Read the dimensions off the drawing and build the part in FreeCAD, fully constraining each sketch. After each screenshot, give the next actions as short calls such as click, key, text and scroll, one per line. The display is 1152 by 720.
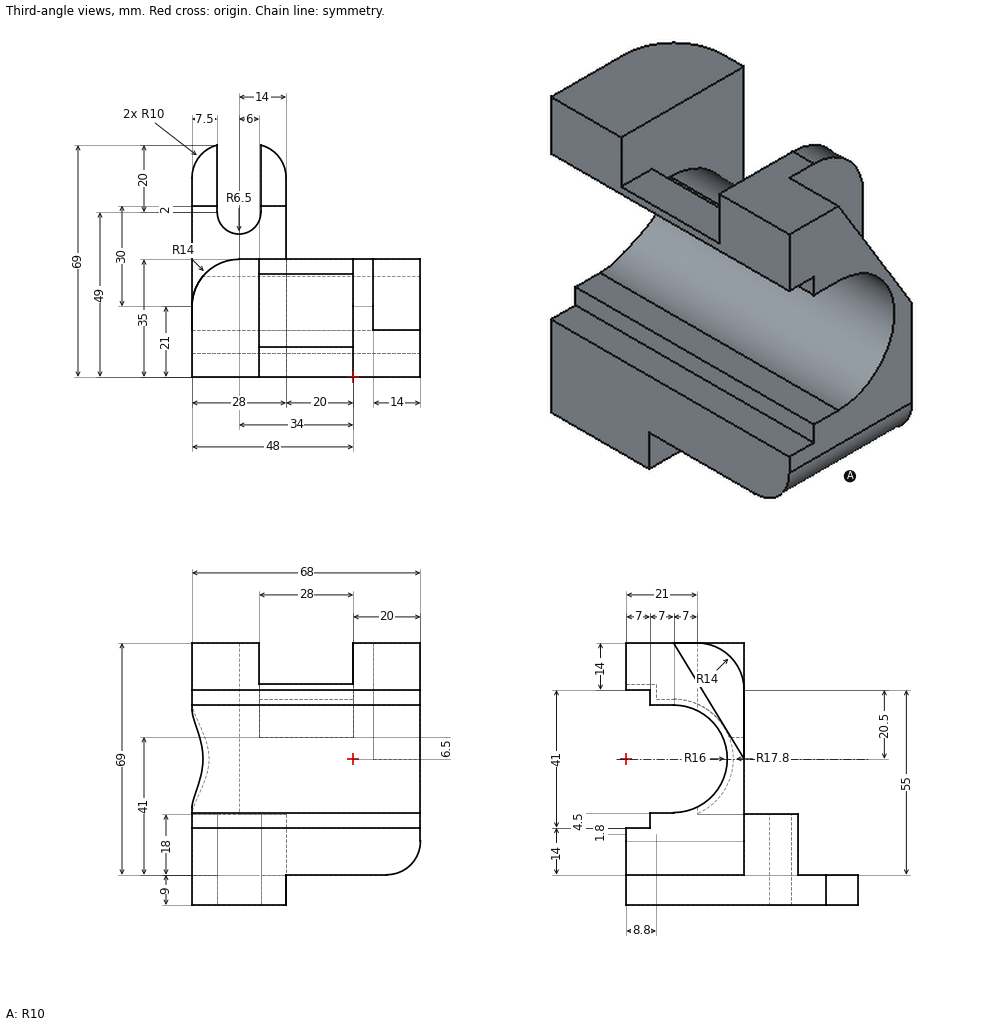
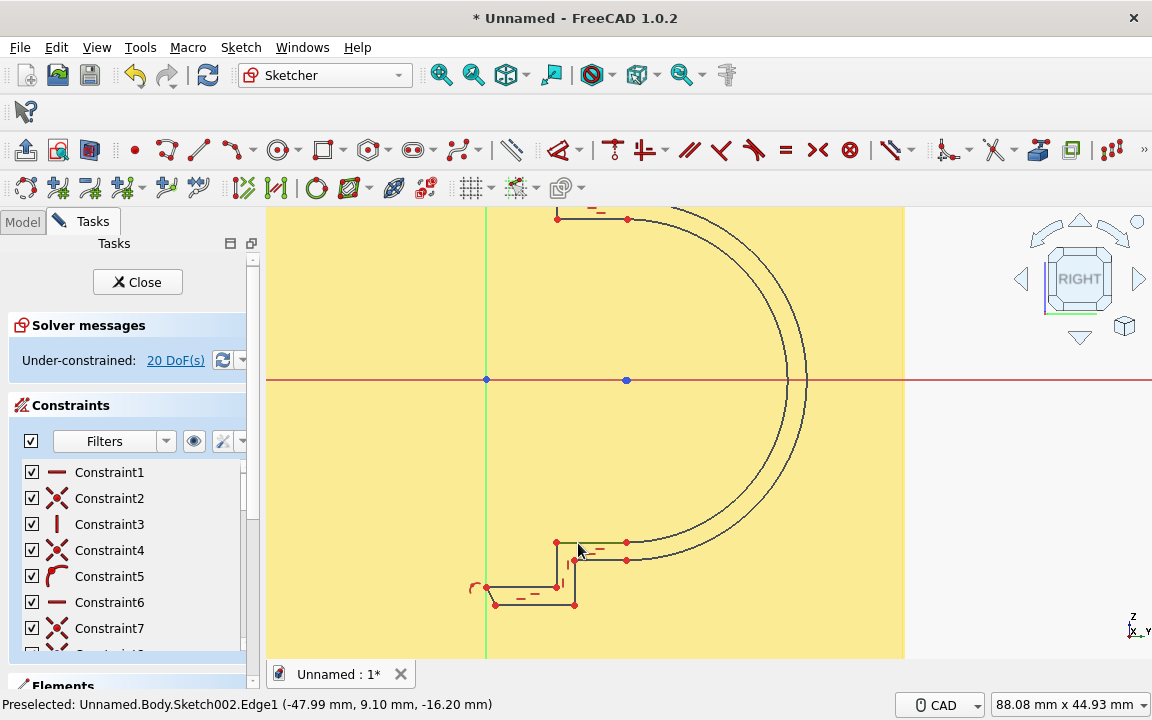
click(757, 476)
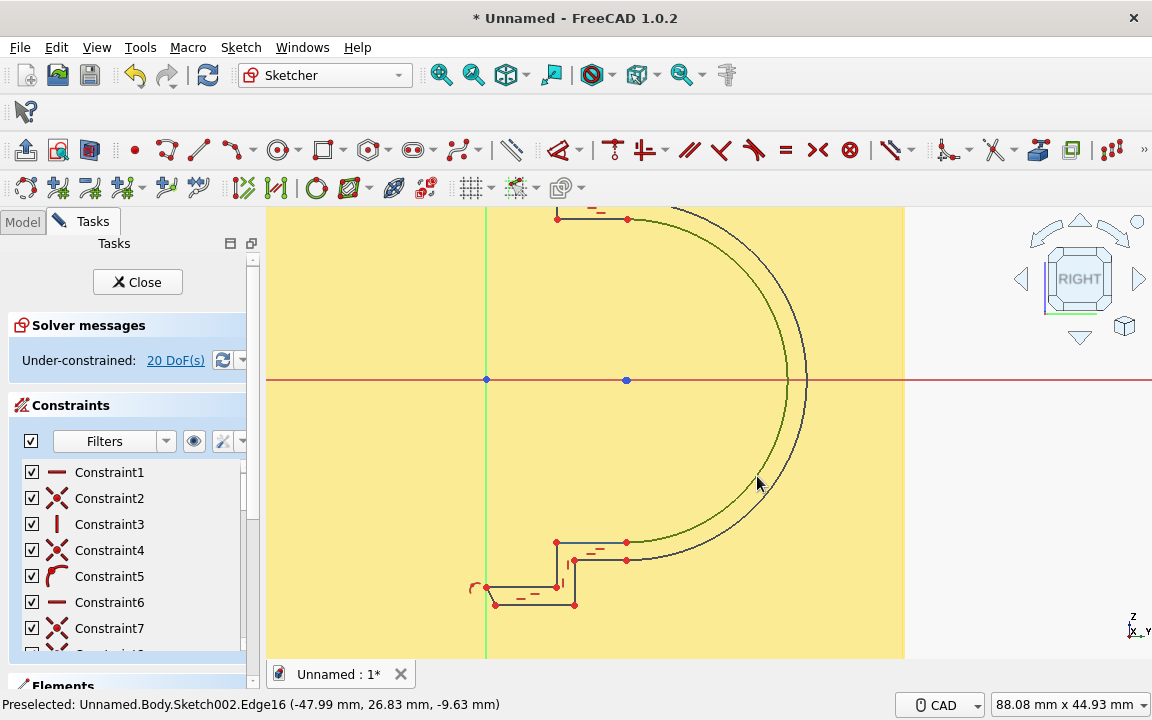
key(t)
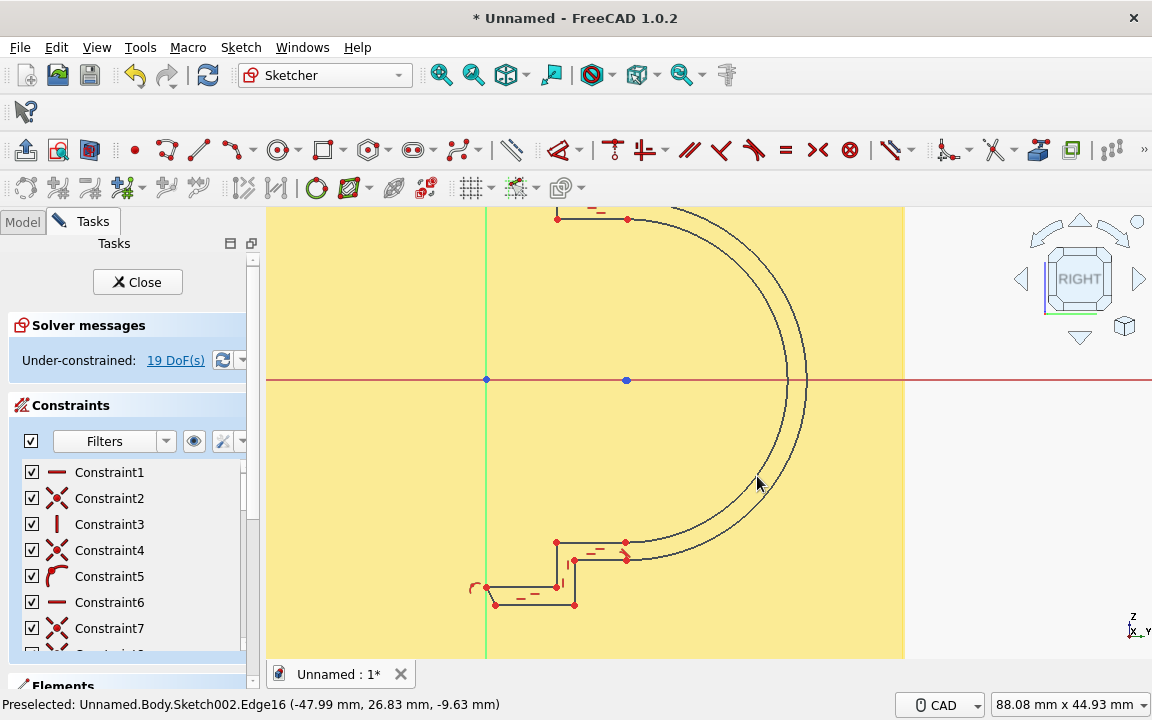
click(590, 560)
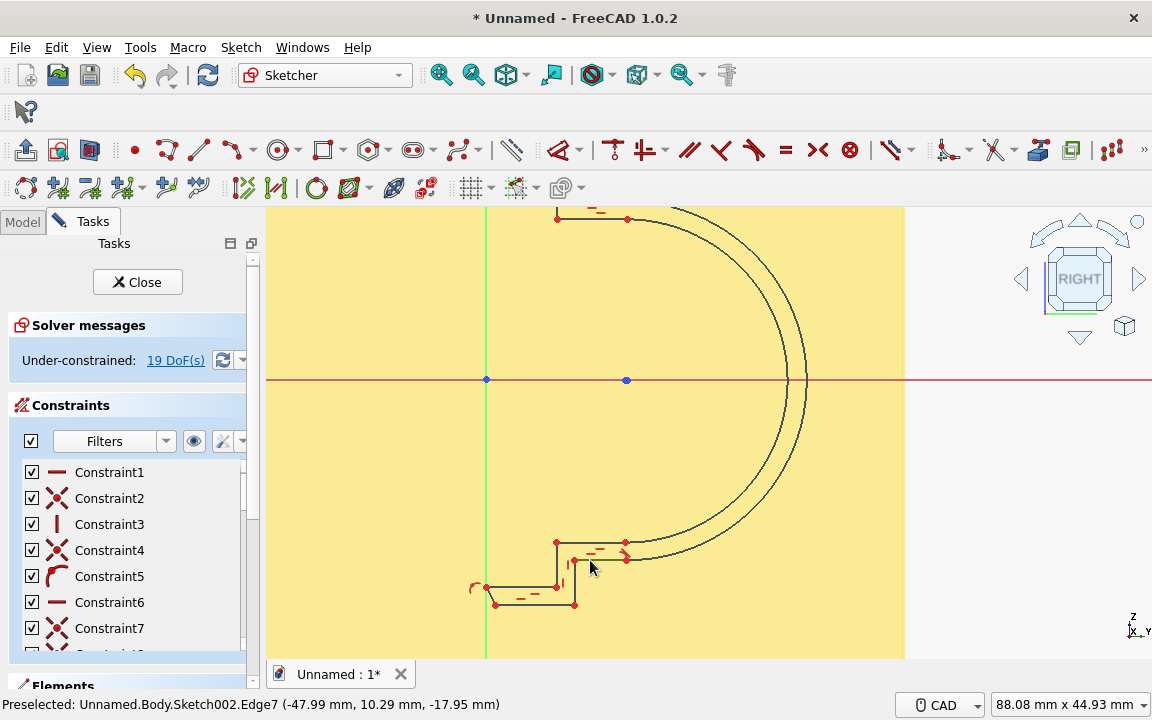
click(772, 487)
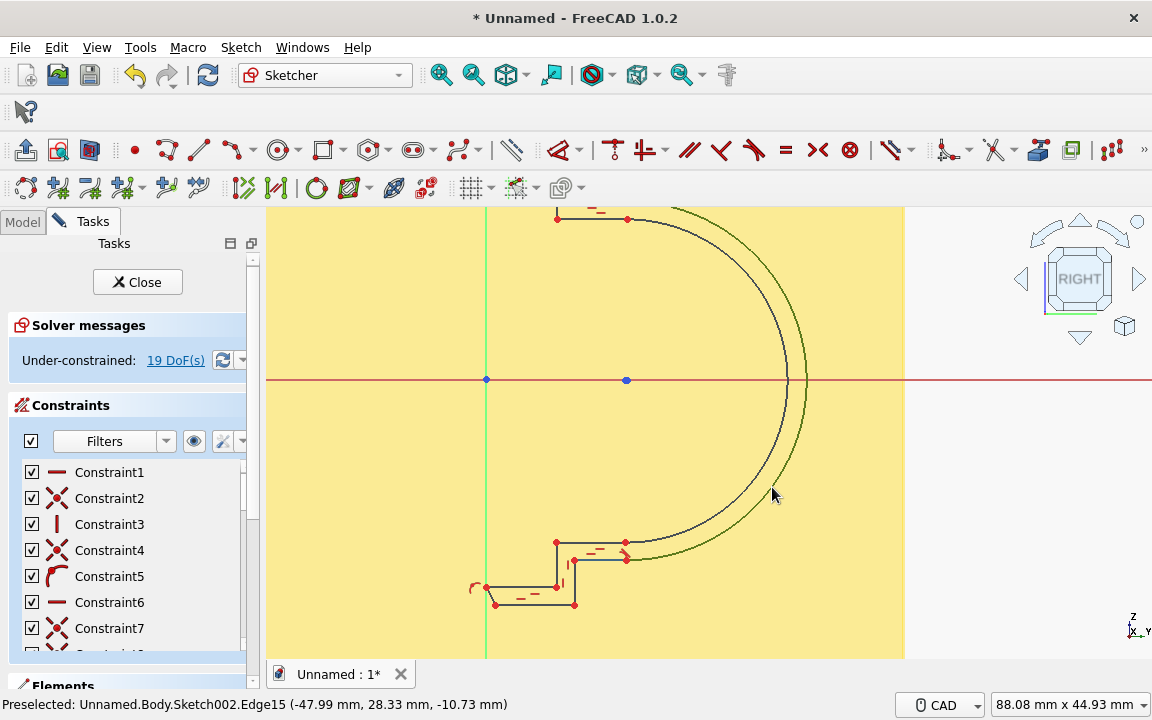
click(754, 150)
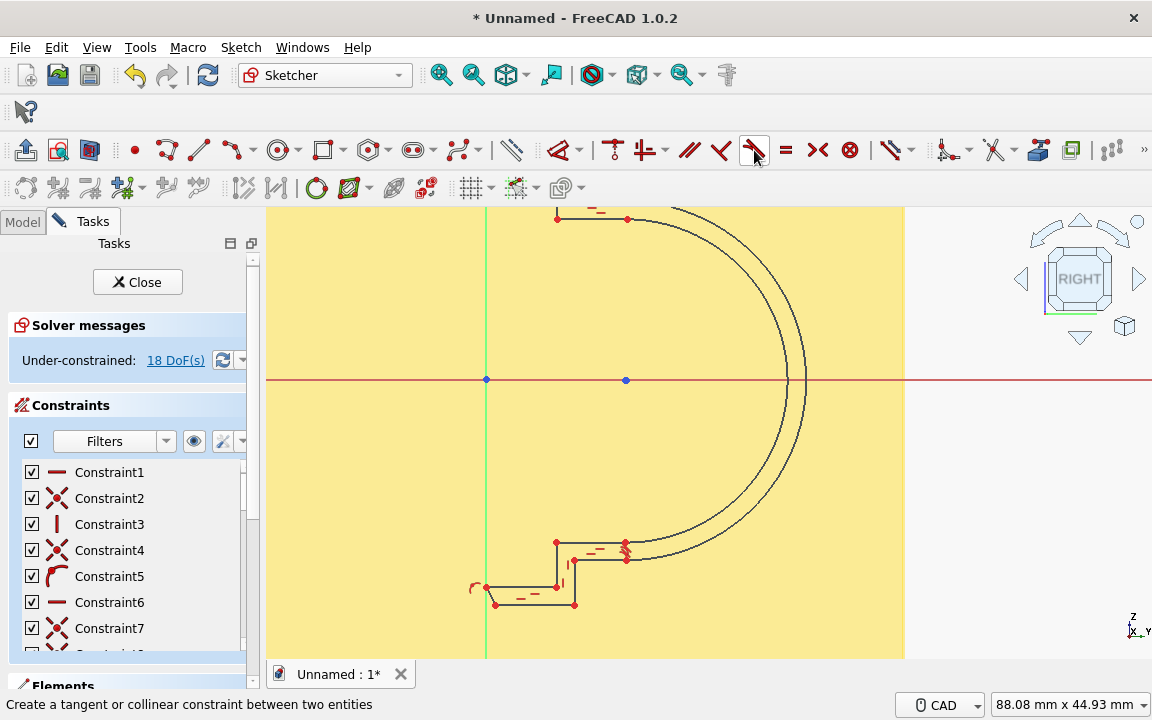
scroll(628, 541, down, 2)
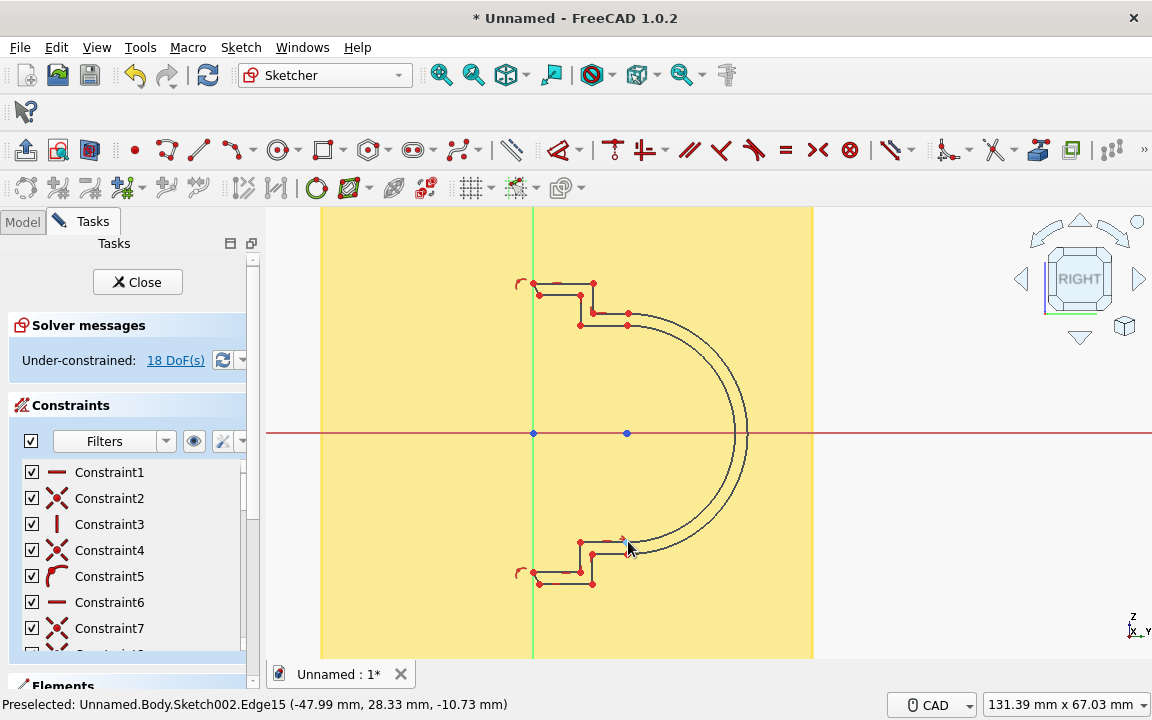
scroll(617, 314, up, 2)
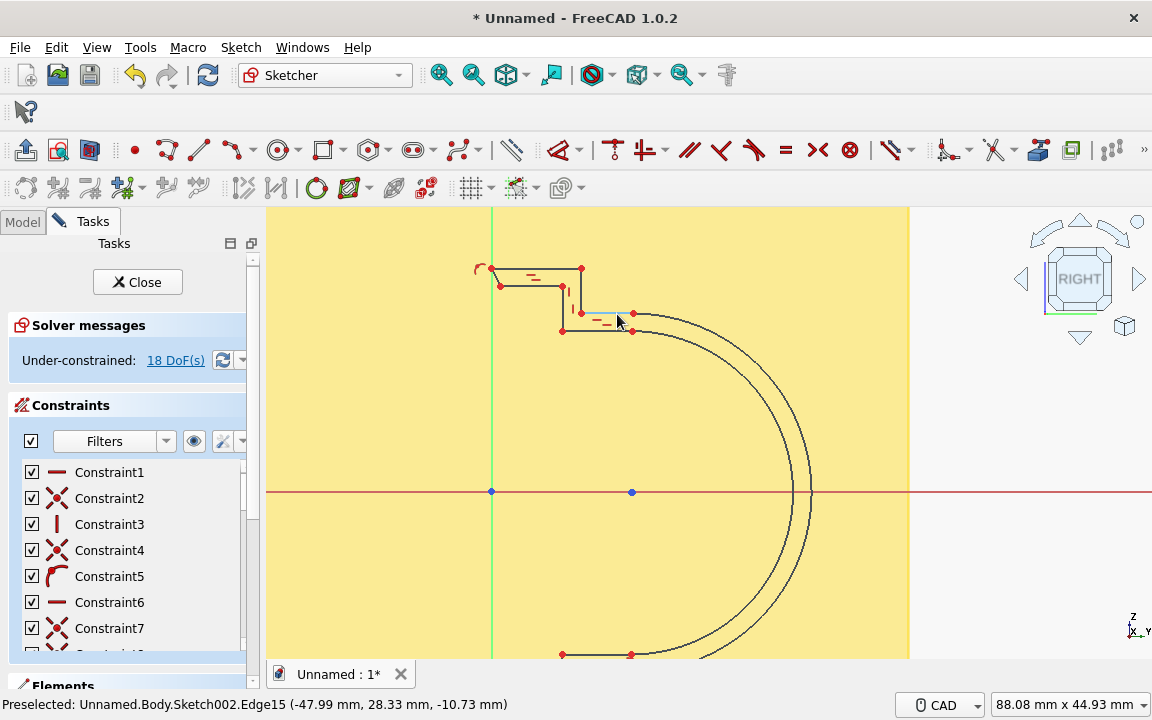
click(618, 313)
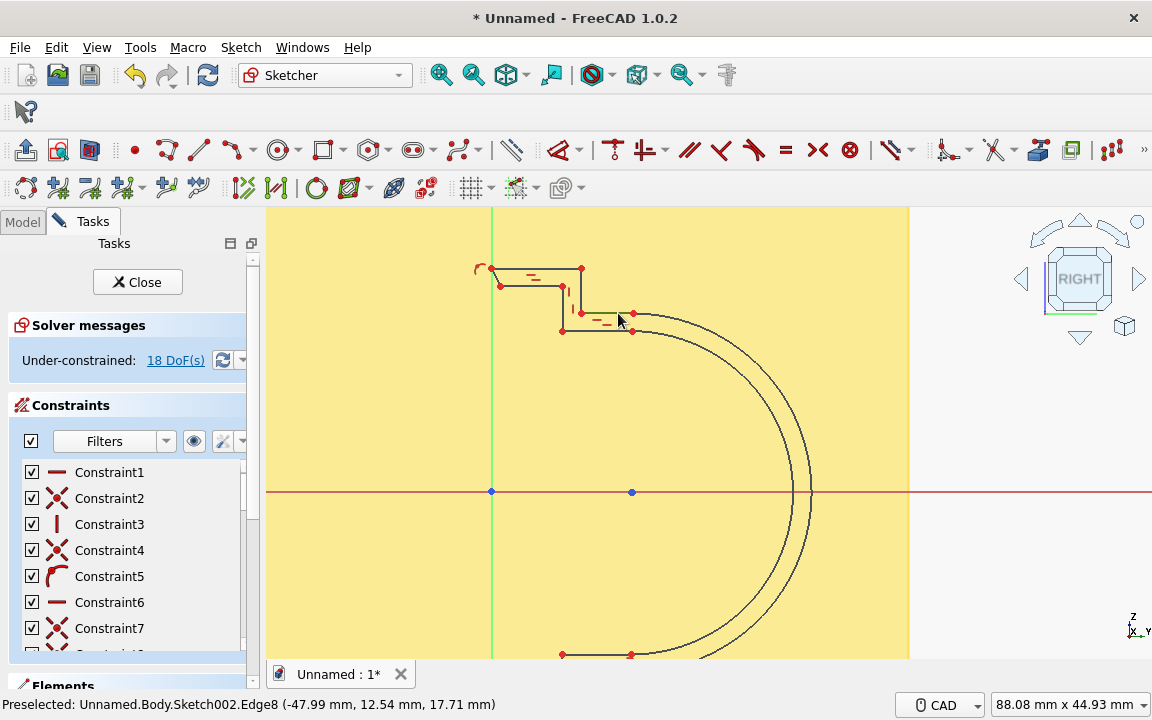
click(777, 598)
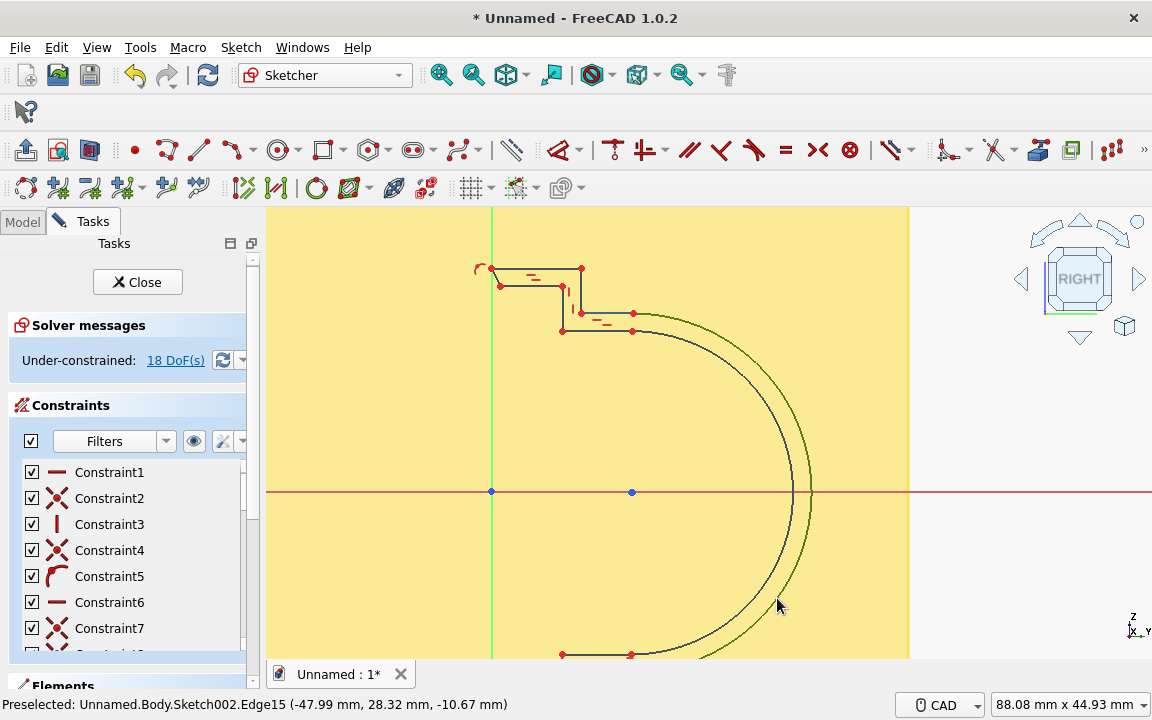
click(754, 150)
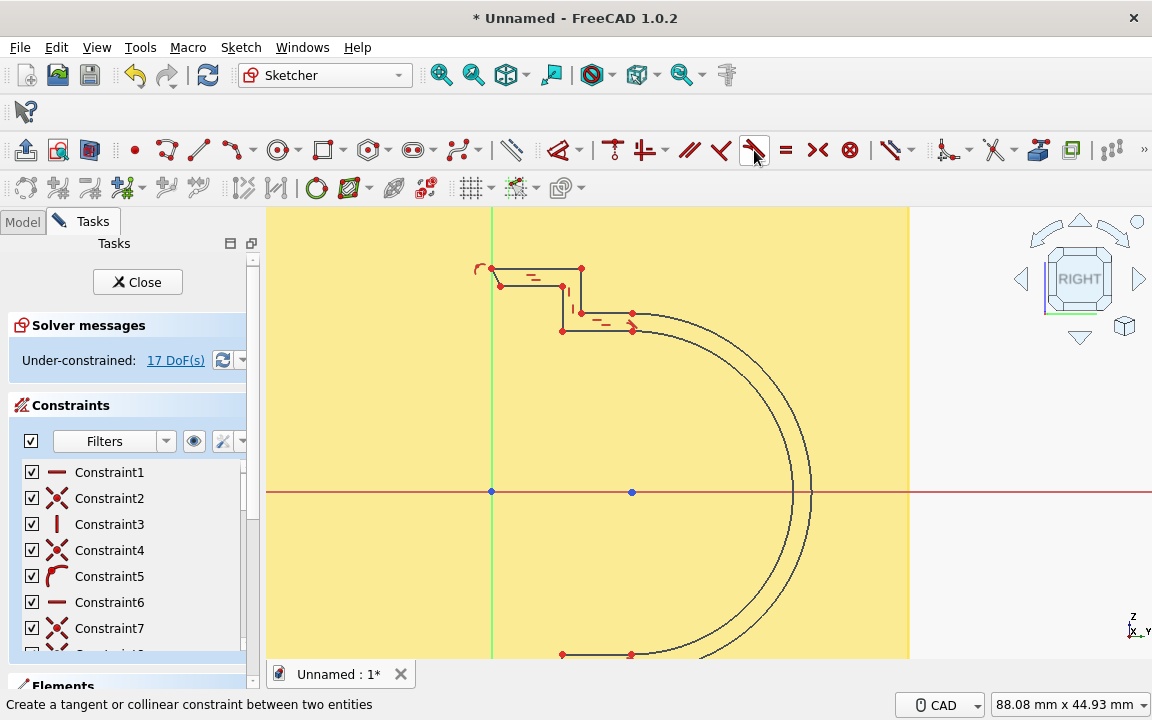
click(584, 331)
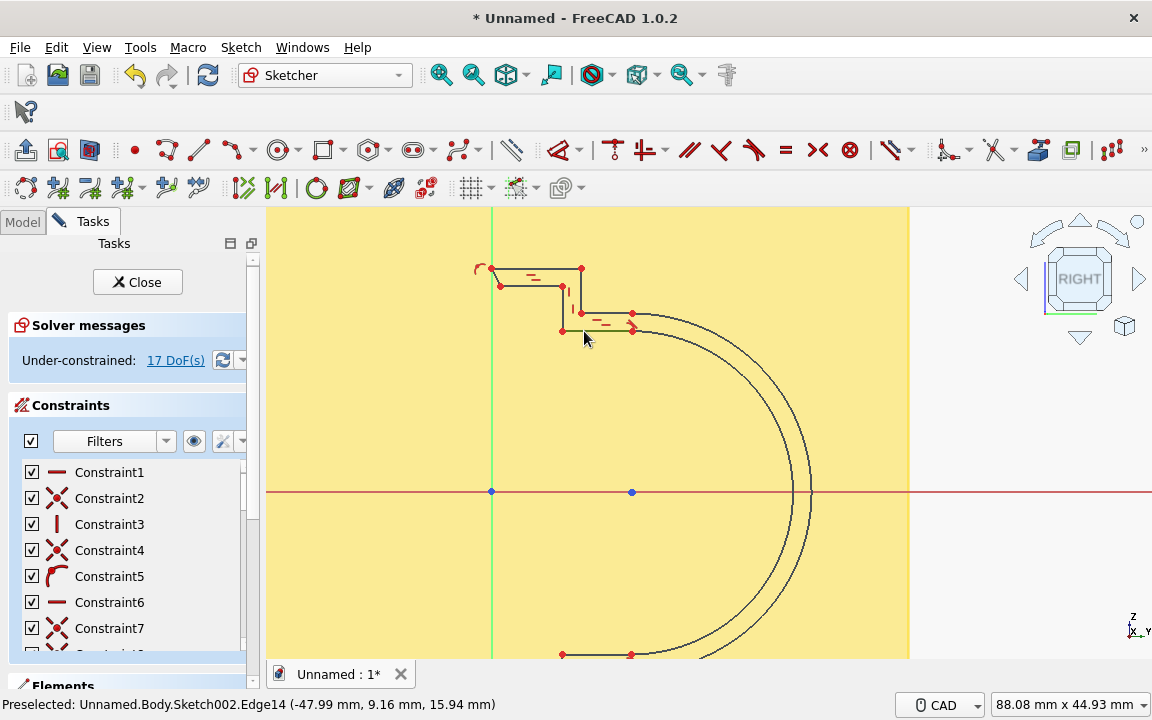
click(762, 588)